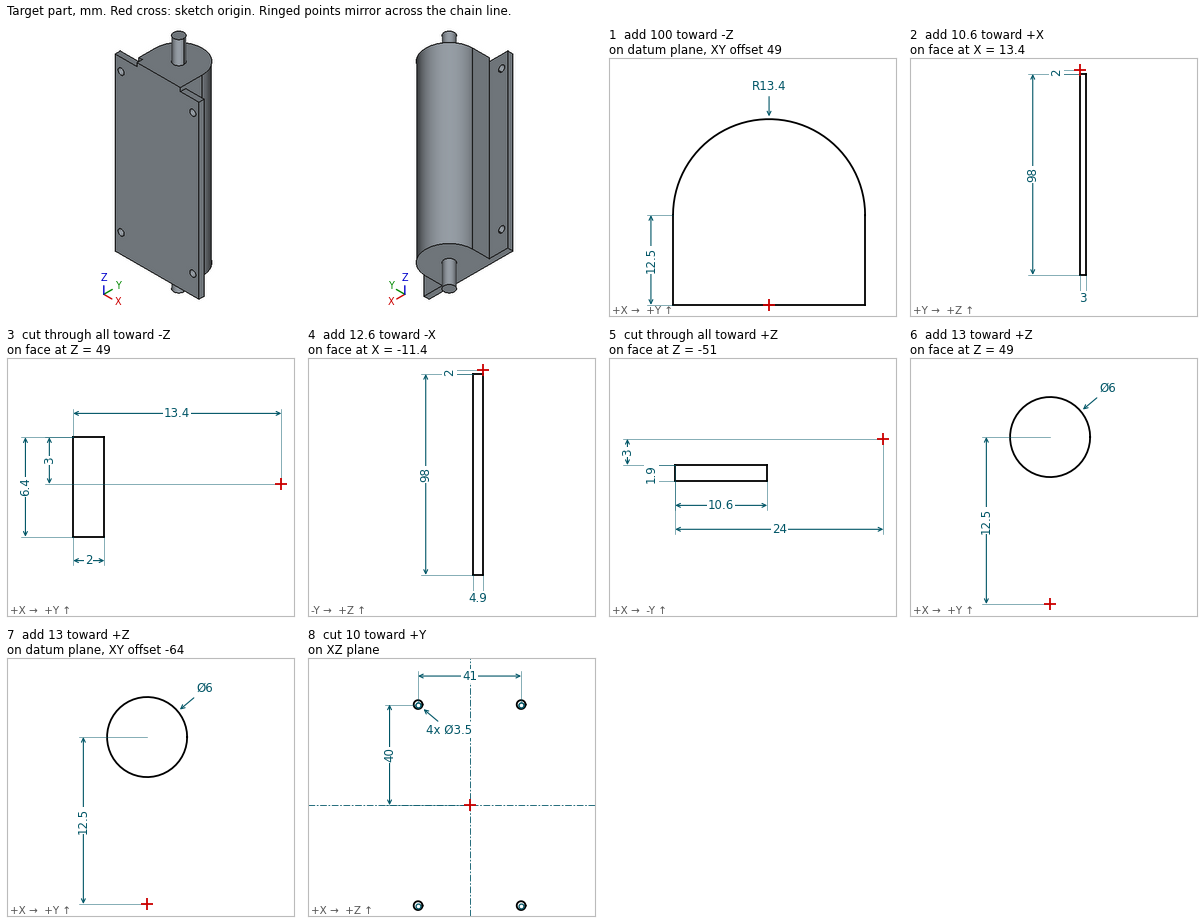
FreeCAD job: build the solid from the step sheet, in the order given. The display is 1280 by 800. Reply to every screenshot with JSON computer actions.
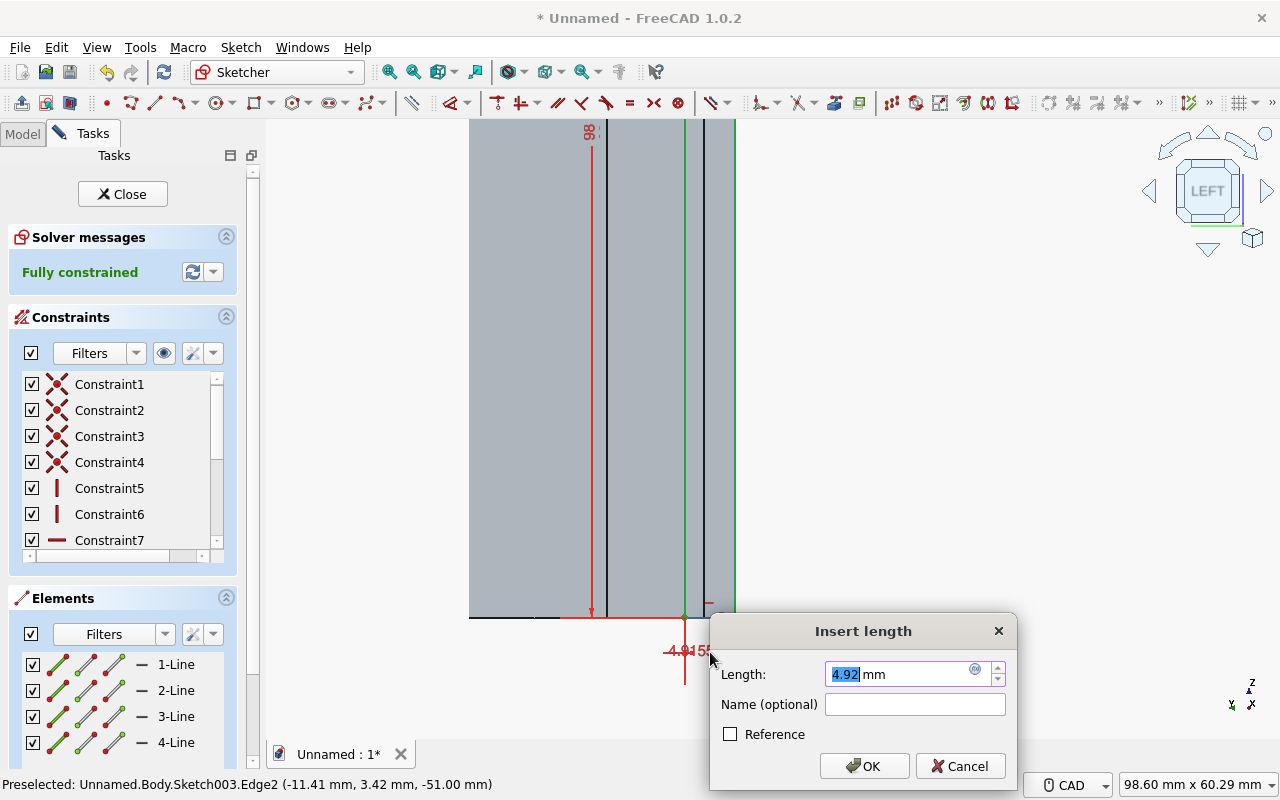
{"action": "type", "text": "4.9"}
{"action": "key", "text": "Return"}
{"action": "key", "text": "Escape"}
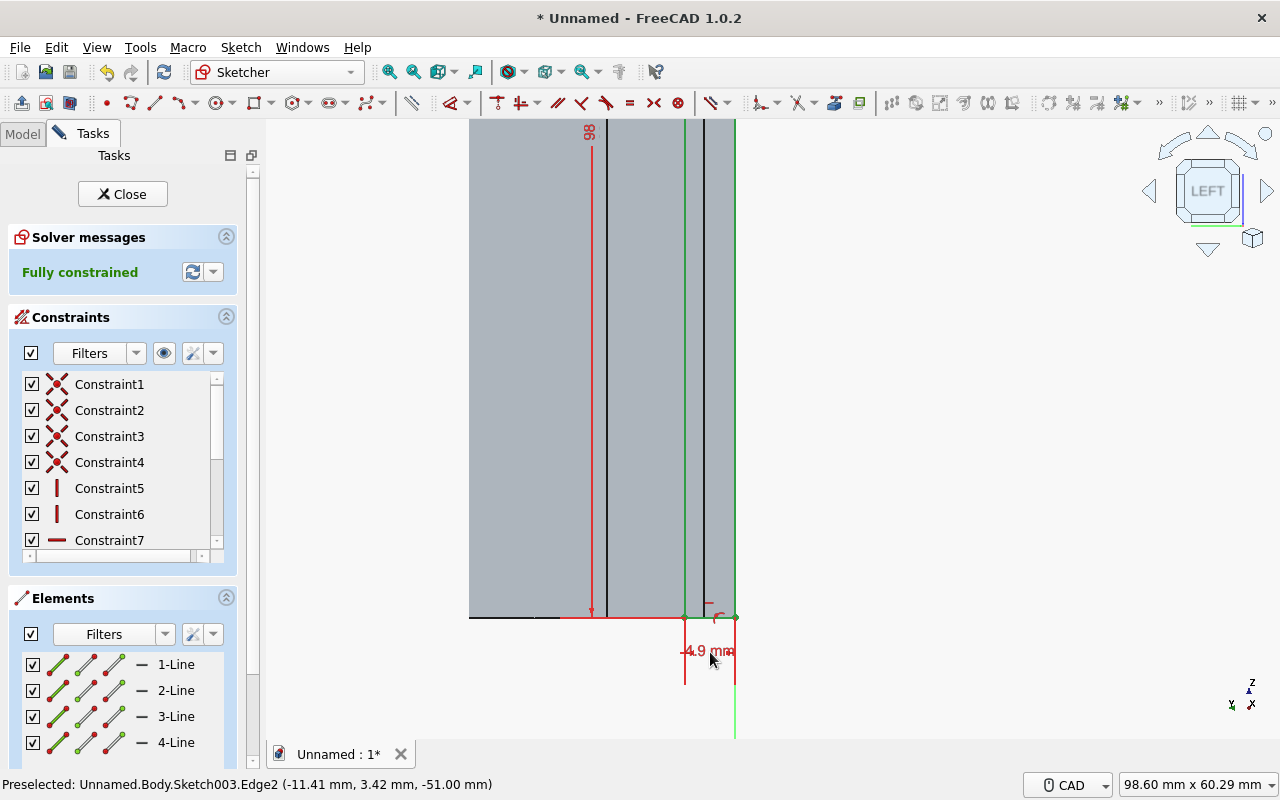
{"action": "left_click", "coordinate": [123, 194]}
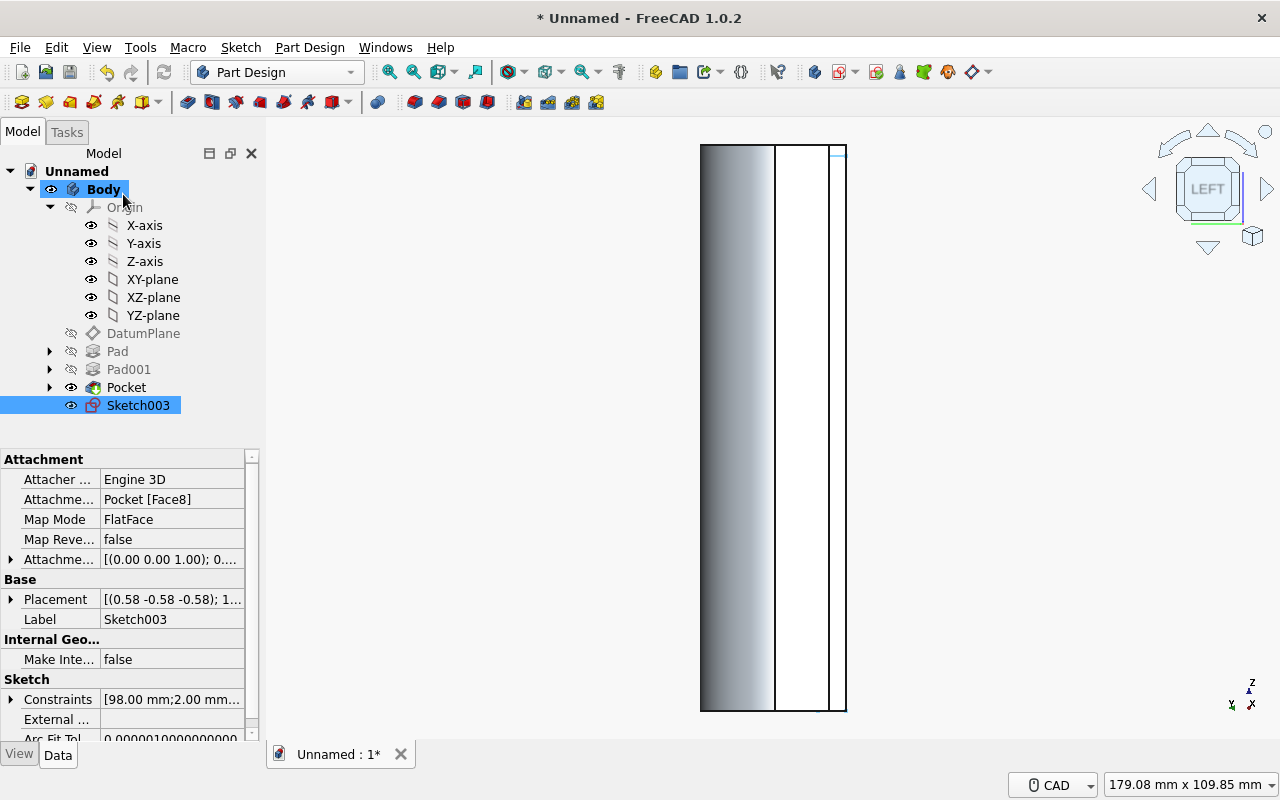
{"action": "left_click", "coordinate": [22, 102]}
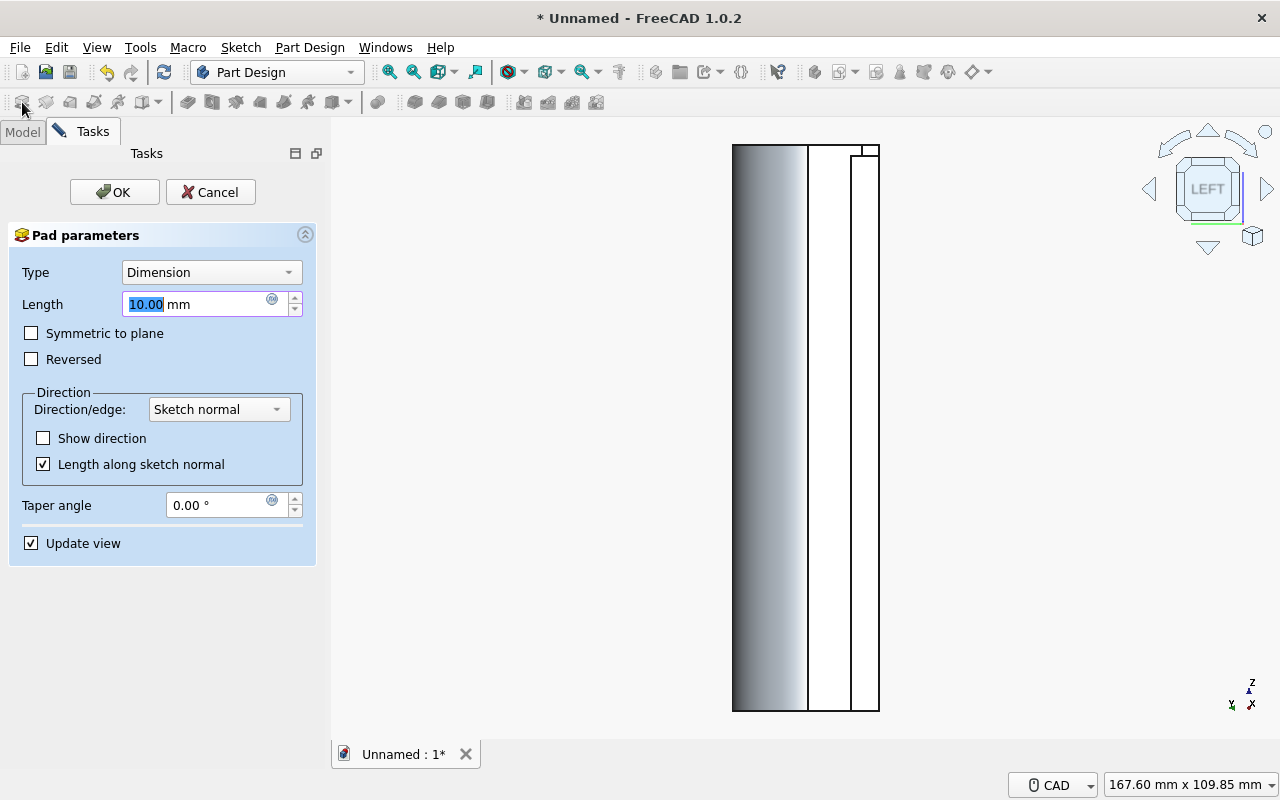
{"action": "type", "text": "12.6"}
{"action": "key", "text": "Tab"}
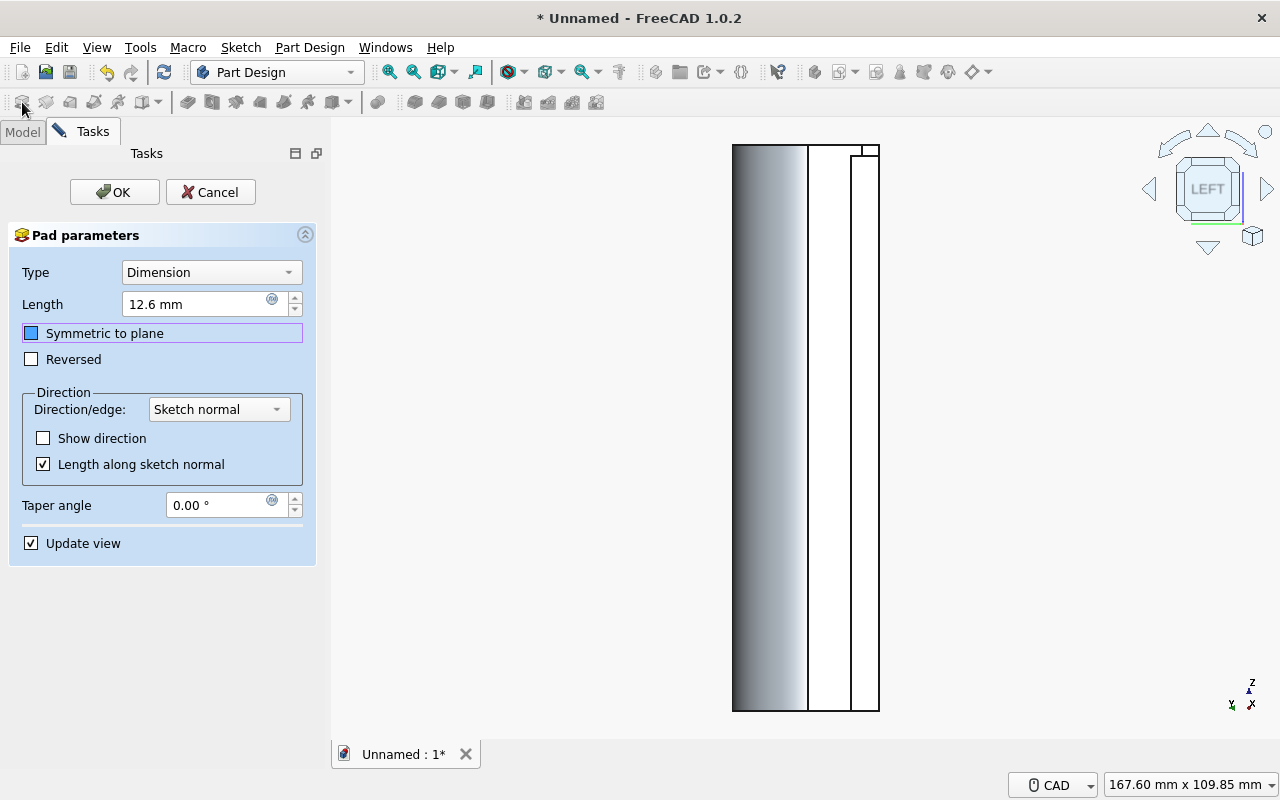
{"action": "left_click", "coordinate": [115, 192]}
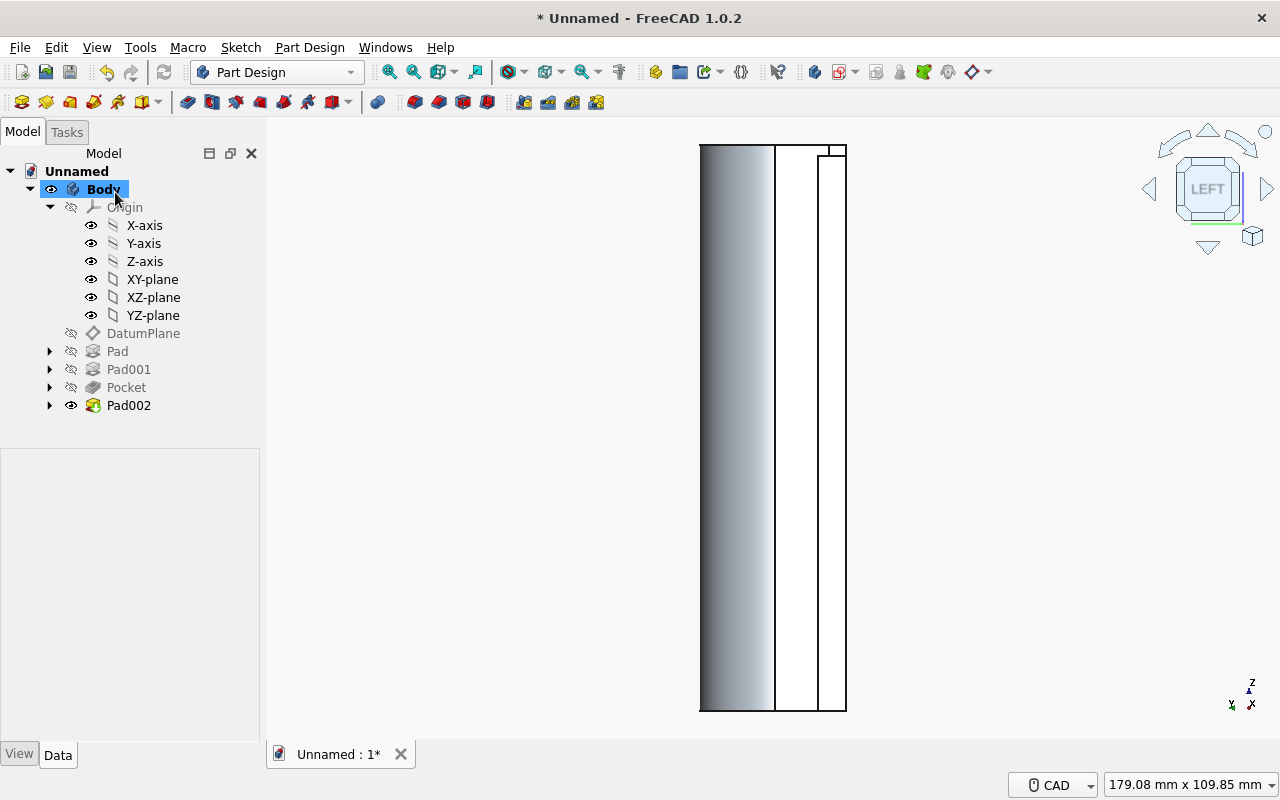
{"action": "key", "text": "5"}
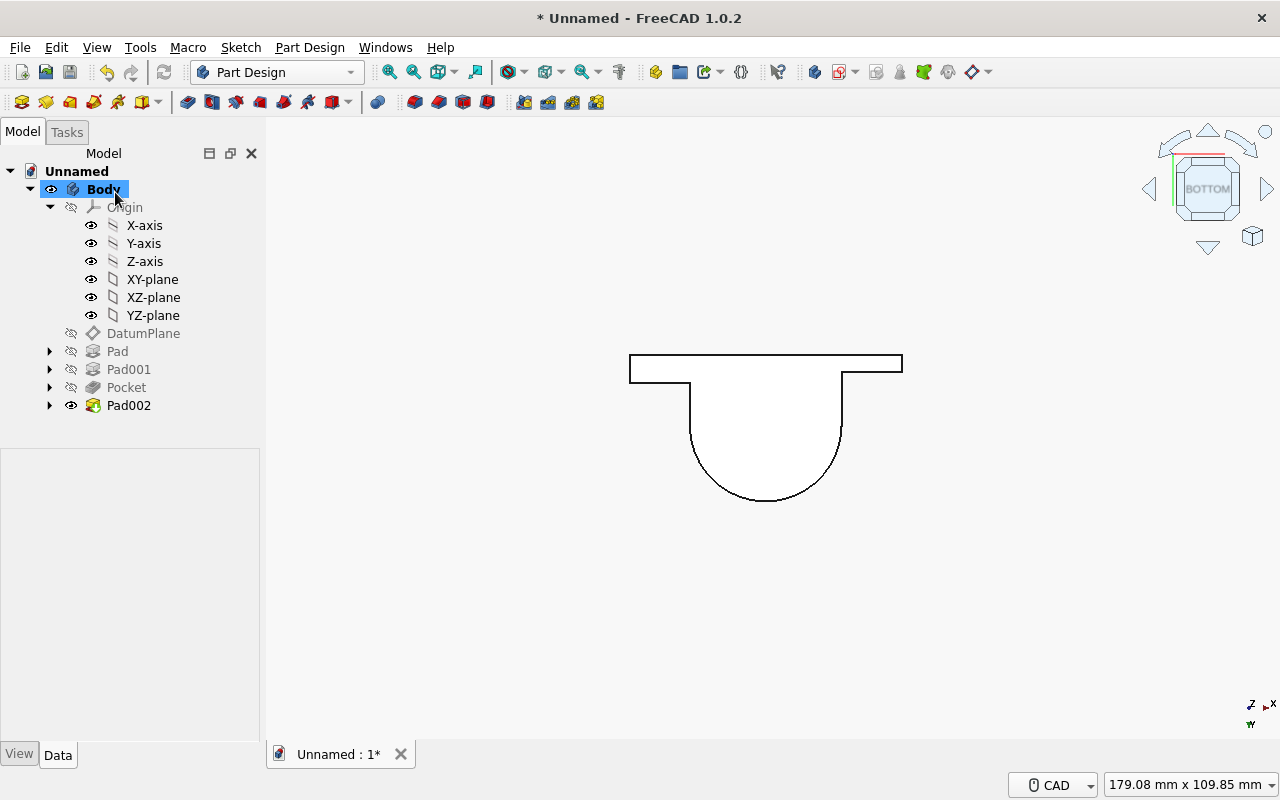
{"action": "left_click", "coordinate": [390, 72]}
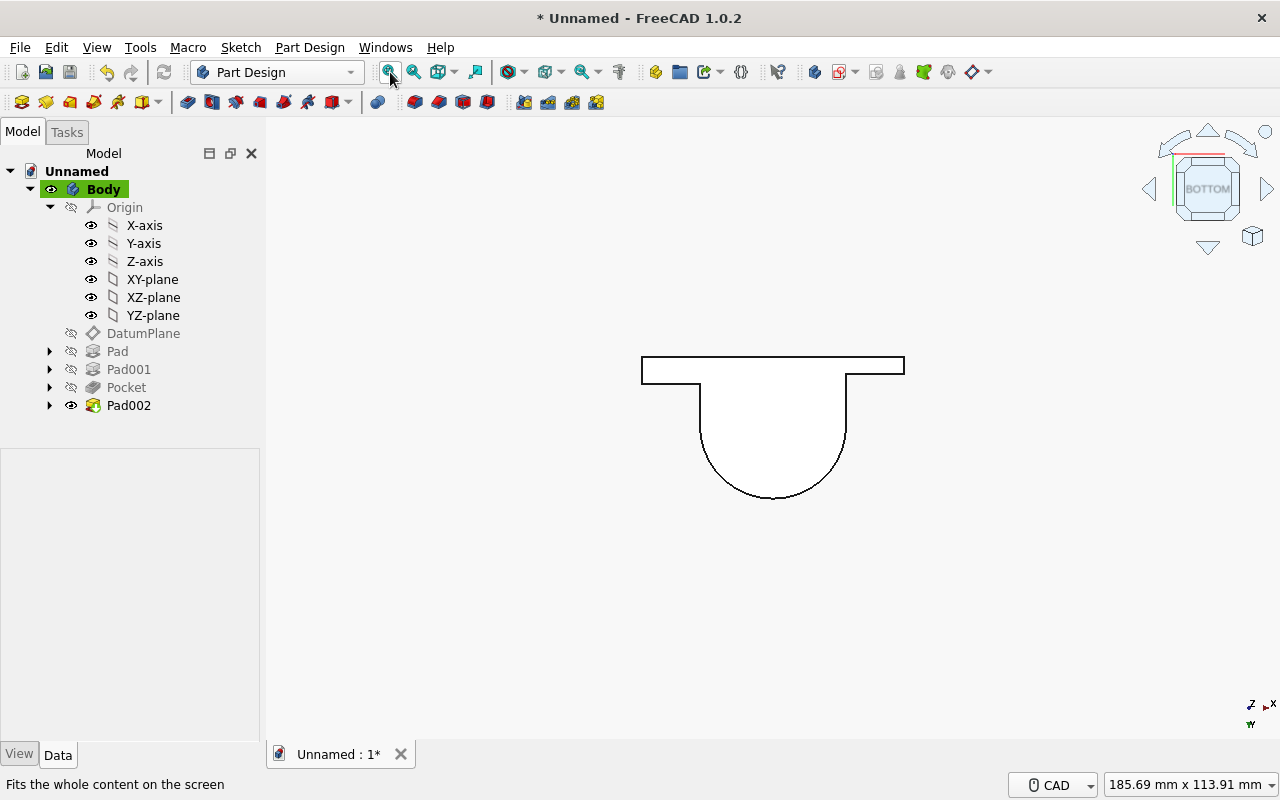
{"action": "left_click", "coordinate": [773, 427]}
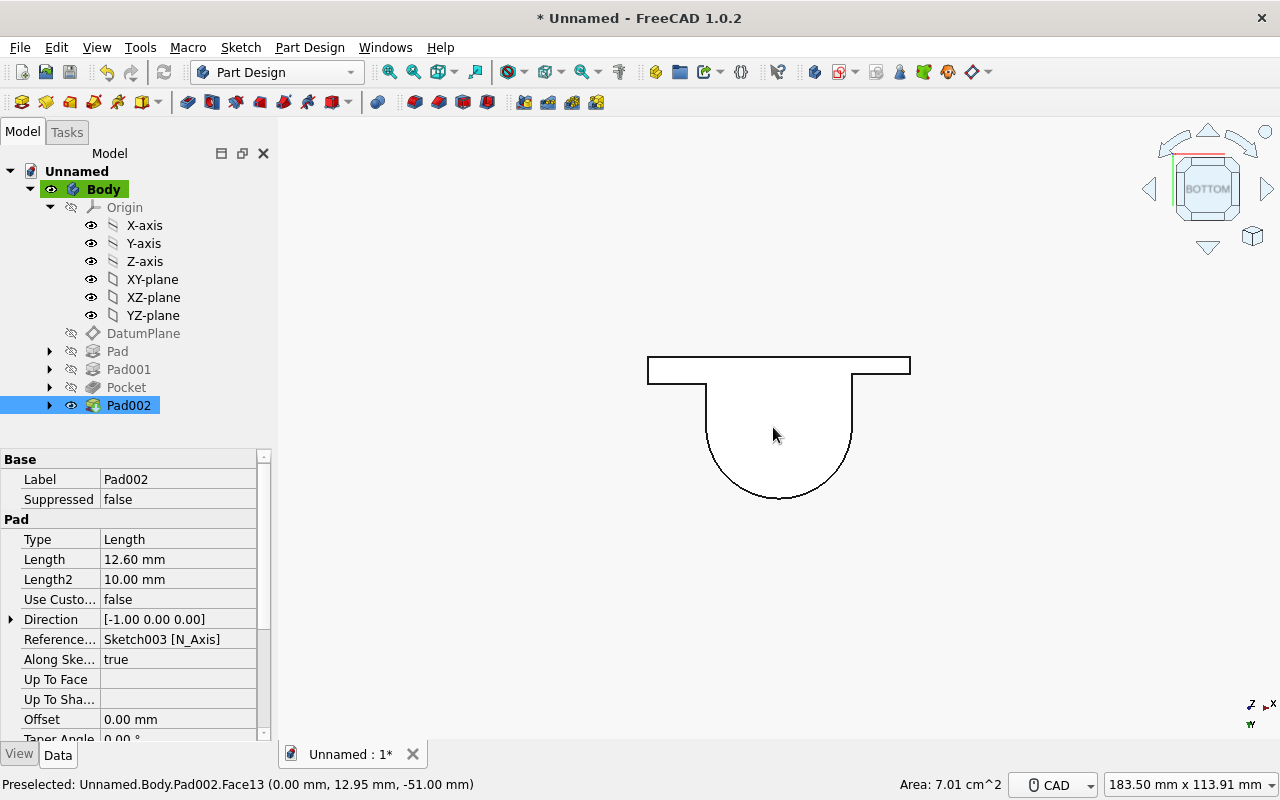
{"action": "left_click", "coordinate": [840, 72]}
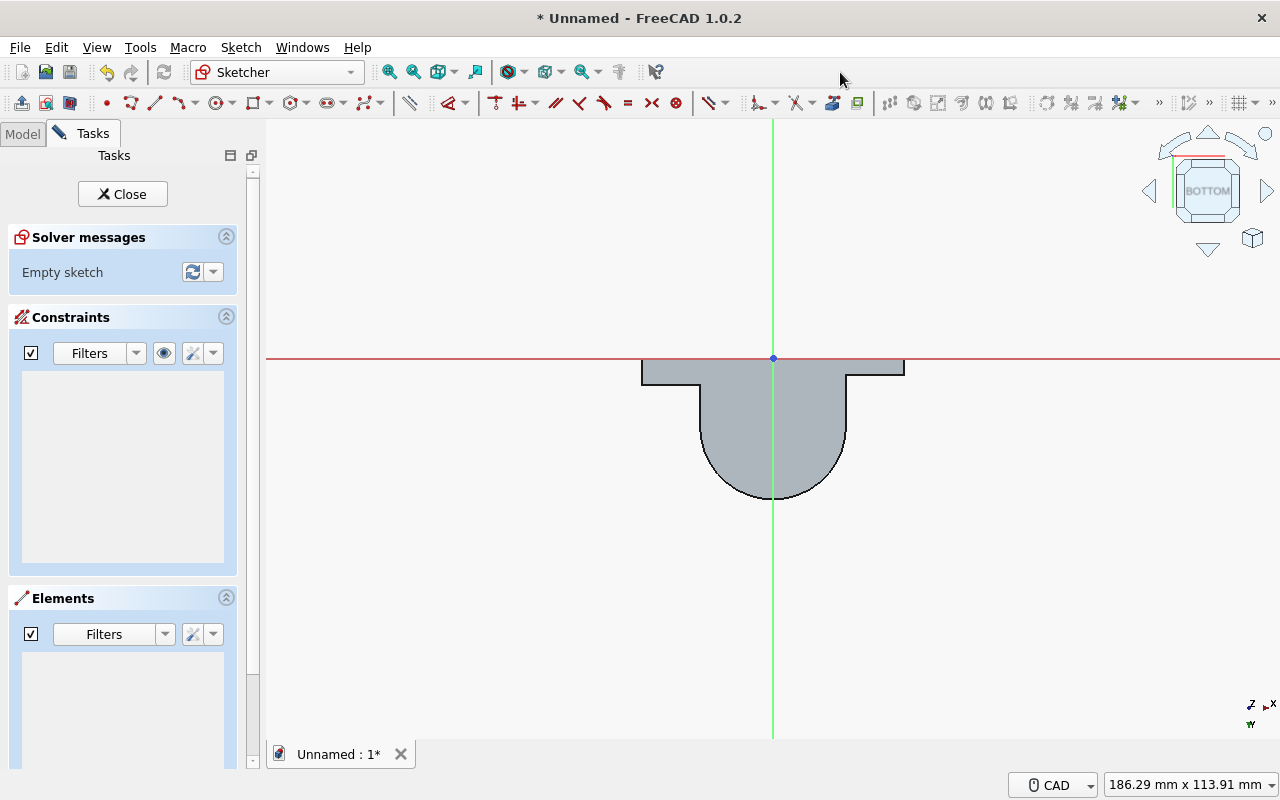
{"action": "scroll", "coordinate": [709, 353], "scroll_direction": "up", "scroll_amount": 7}